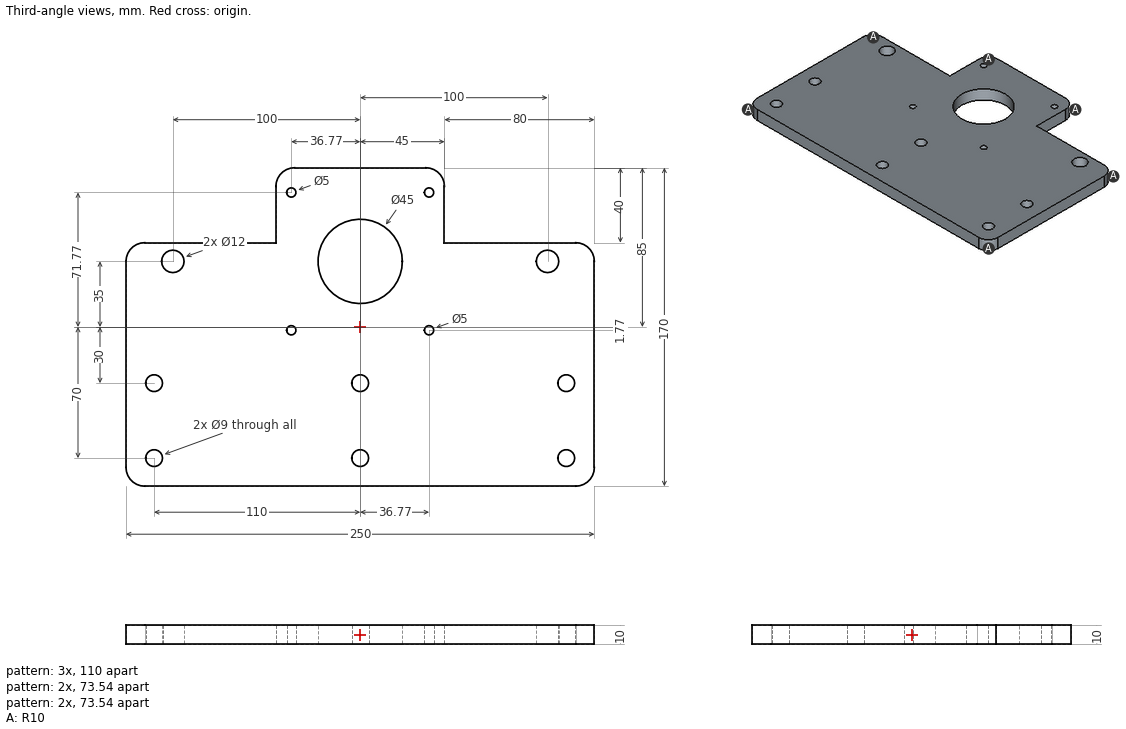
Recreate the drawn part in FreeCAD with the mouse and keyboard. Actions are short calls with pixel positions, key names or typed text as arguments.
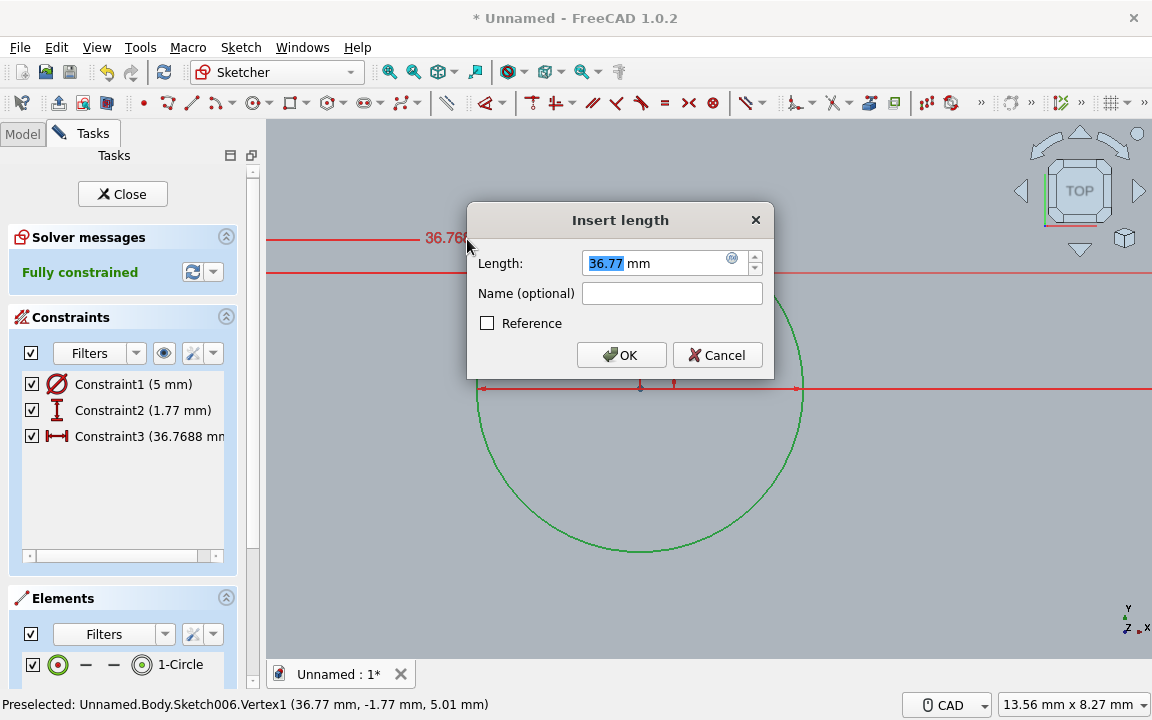
text(36.77)
key(Return)
key(Escape)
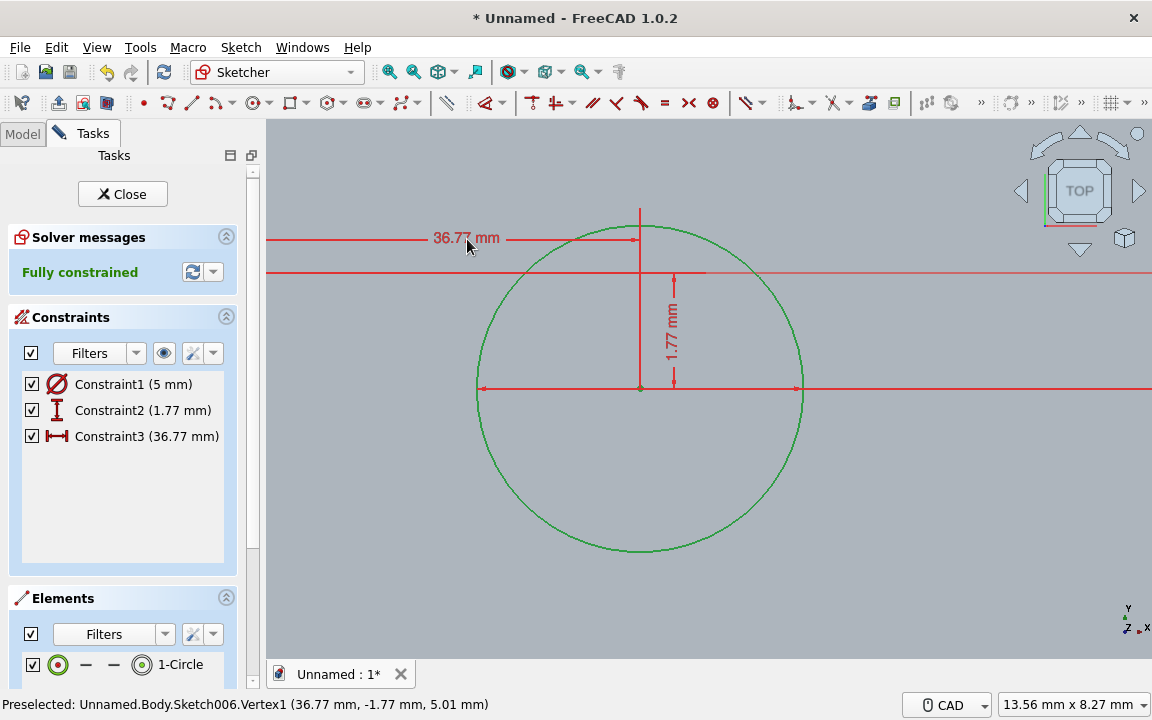
click(123, 194)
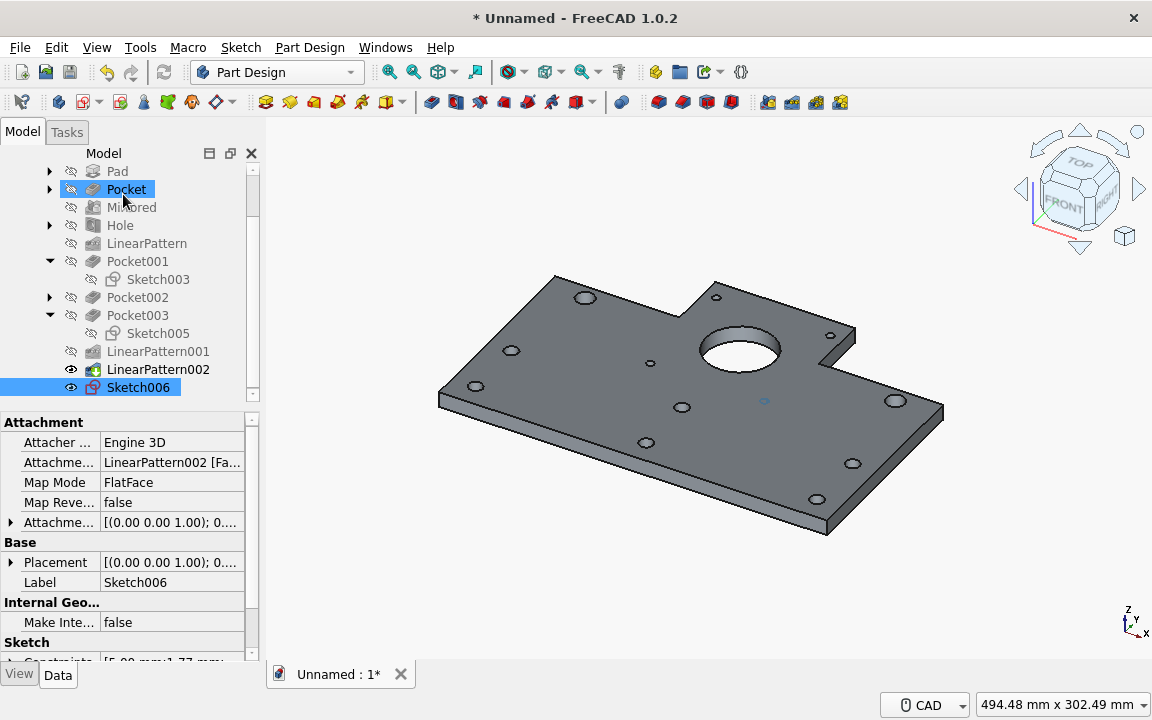
click(432, 102)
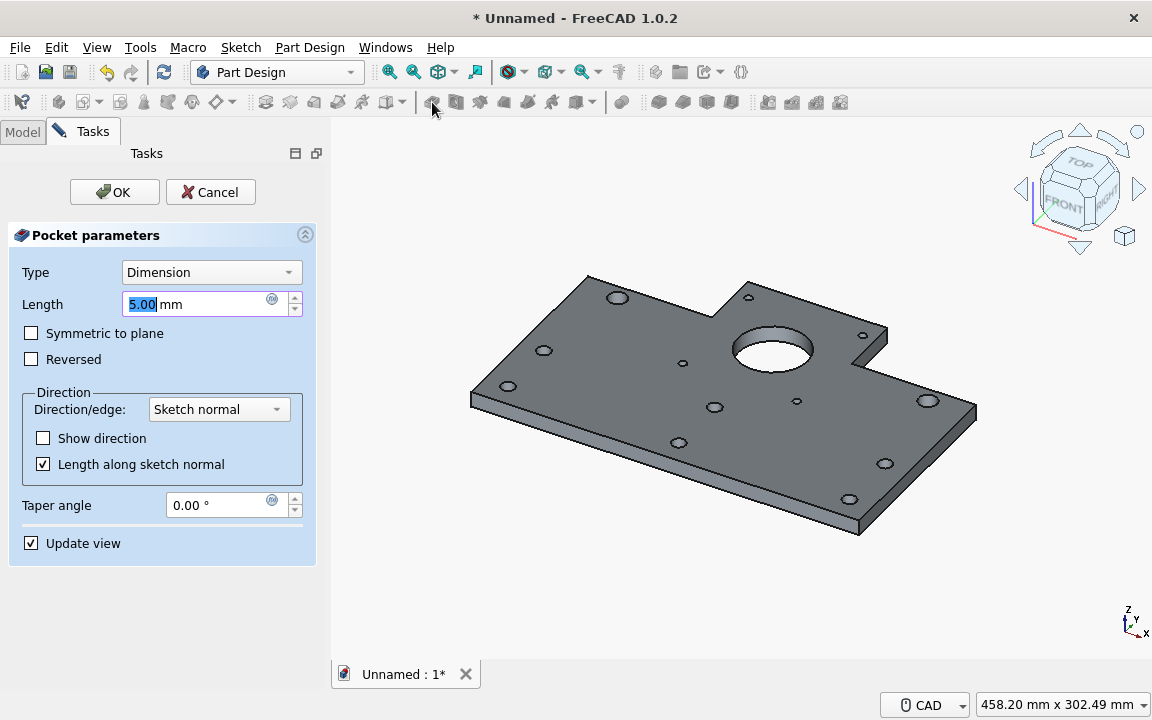
click(212, 272)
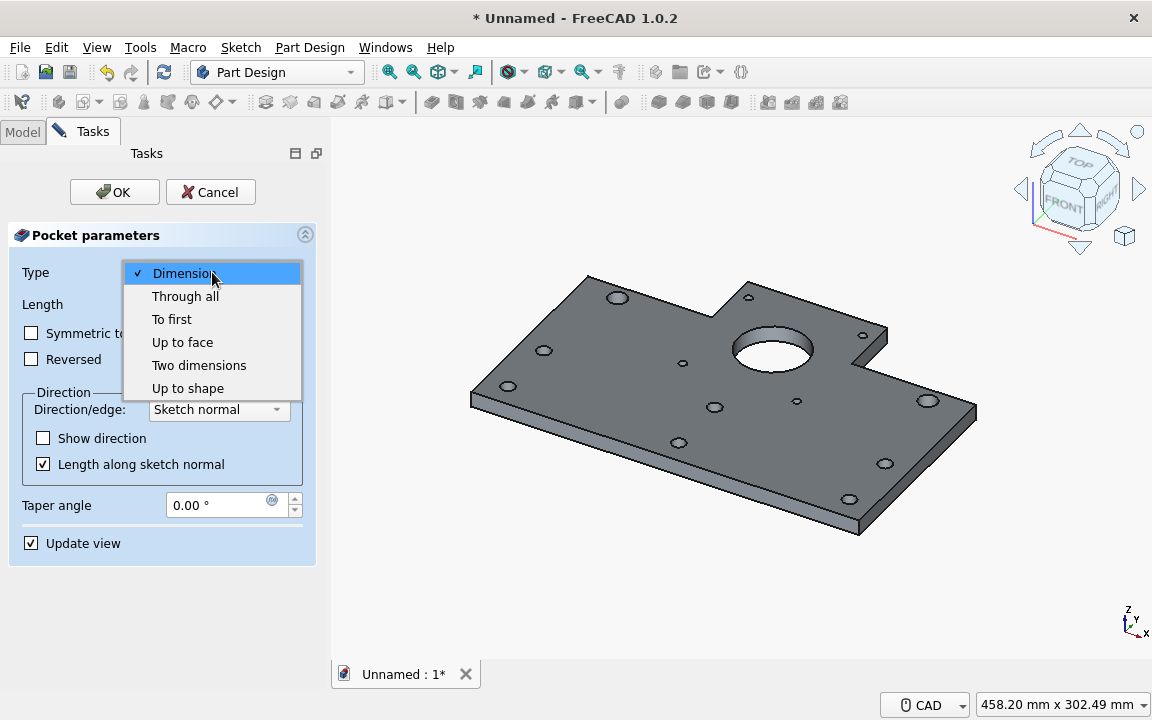
click(212, 296)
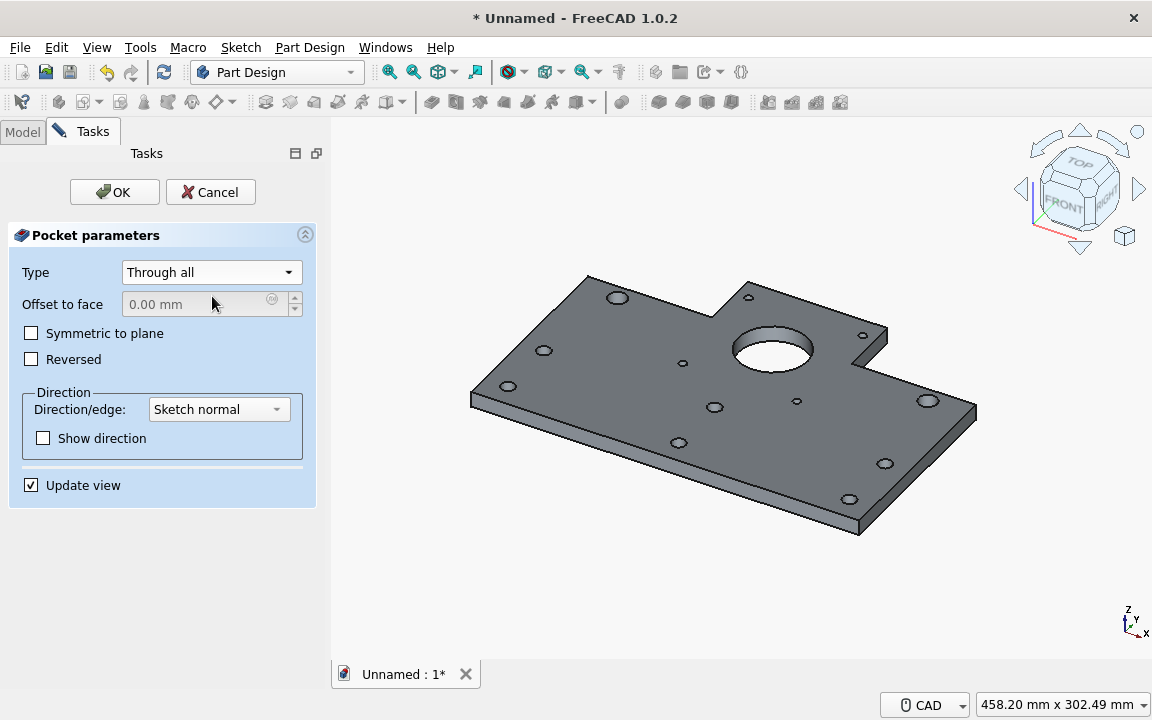
click(115, 192)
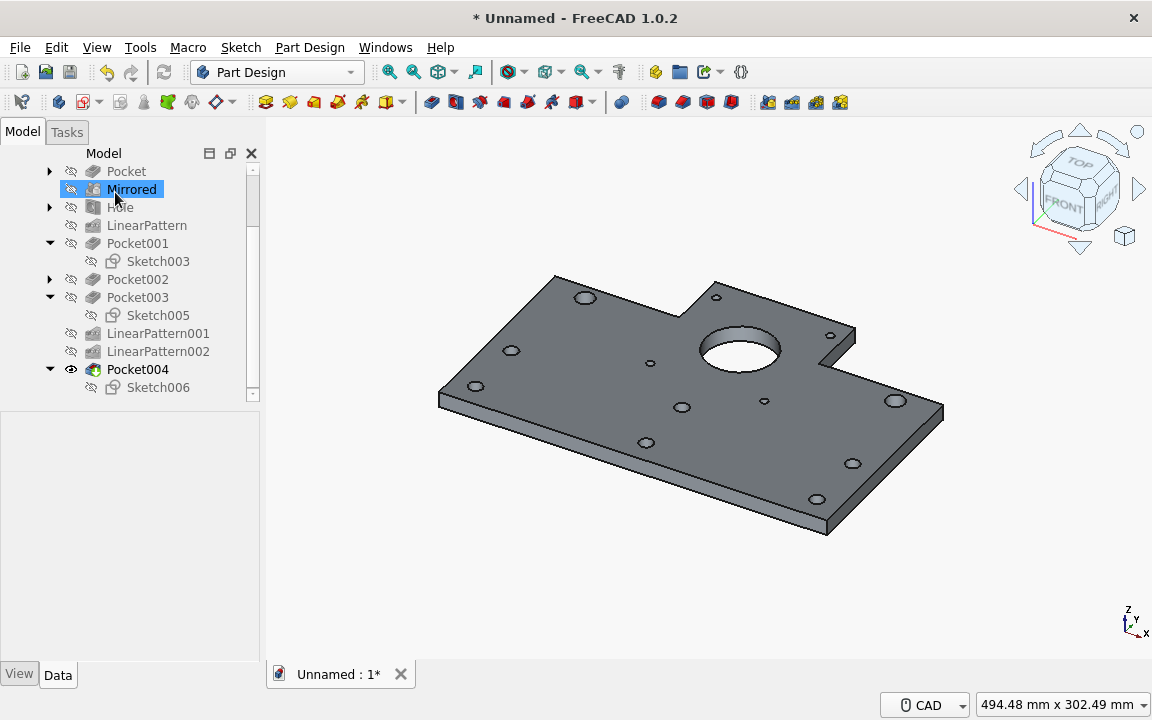
click(827, 527)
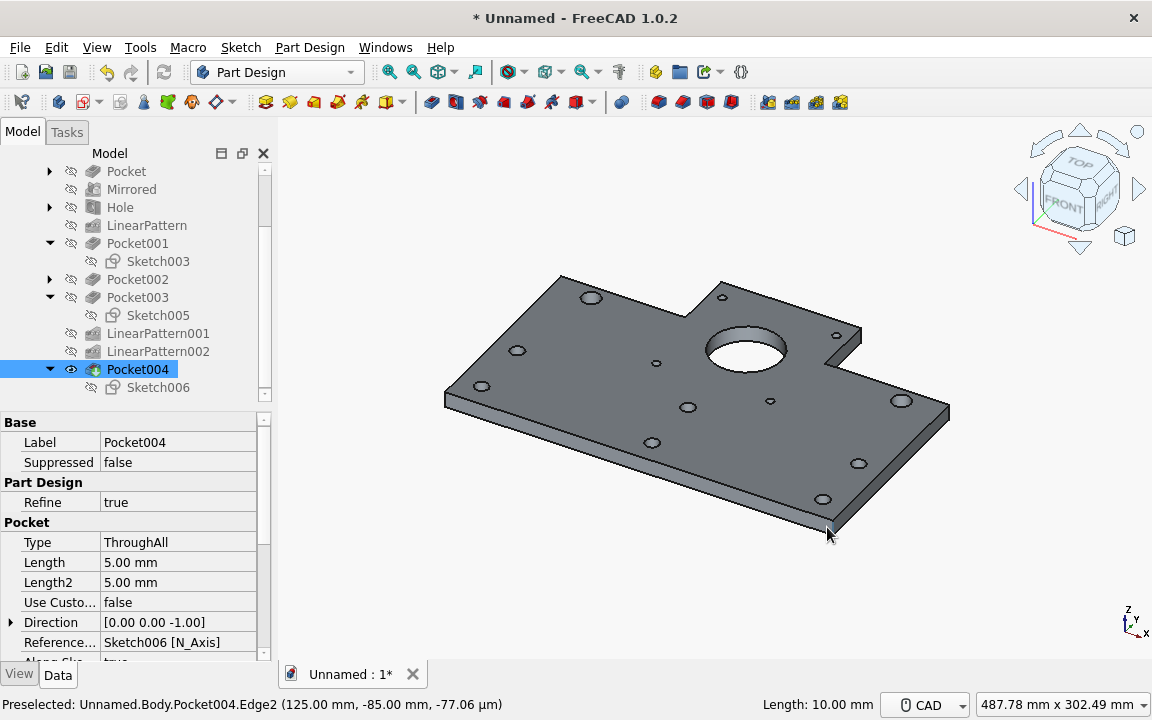
scroll(949, 411, up, 5)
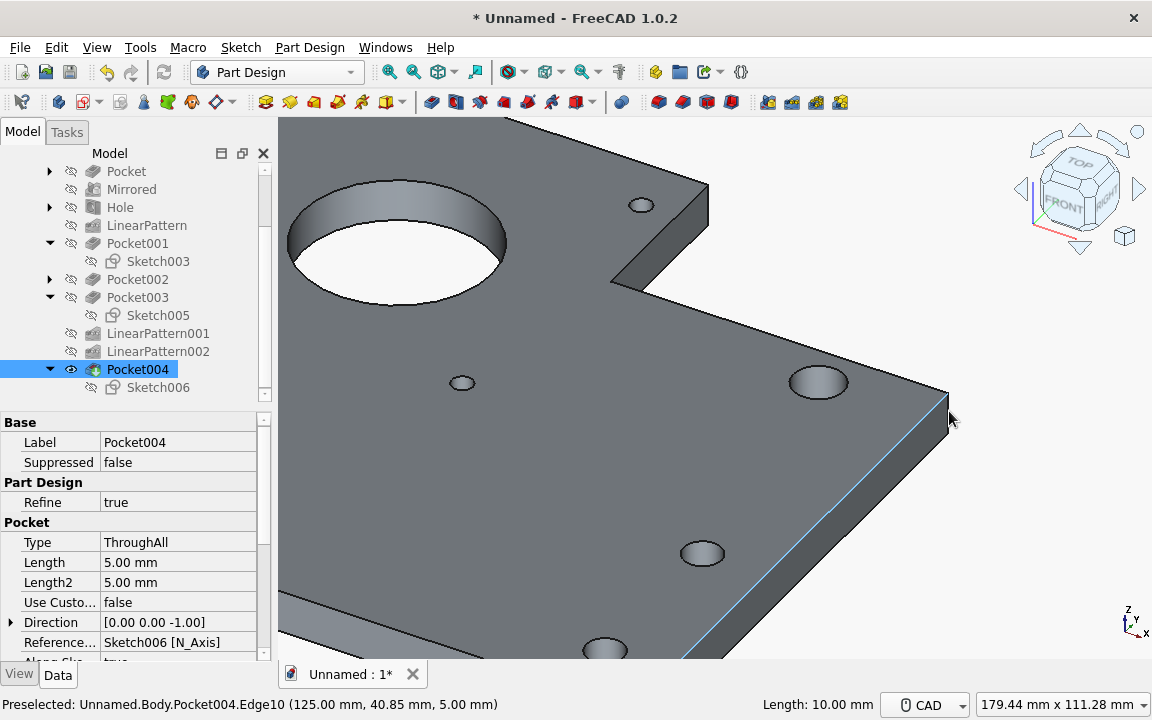
click(390, 72)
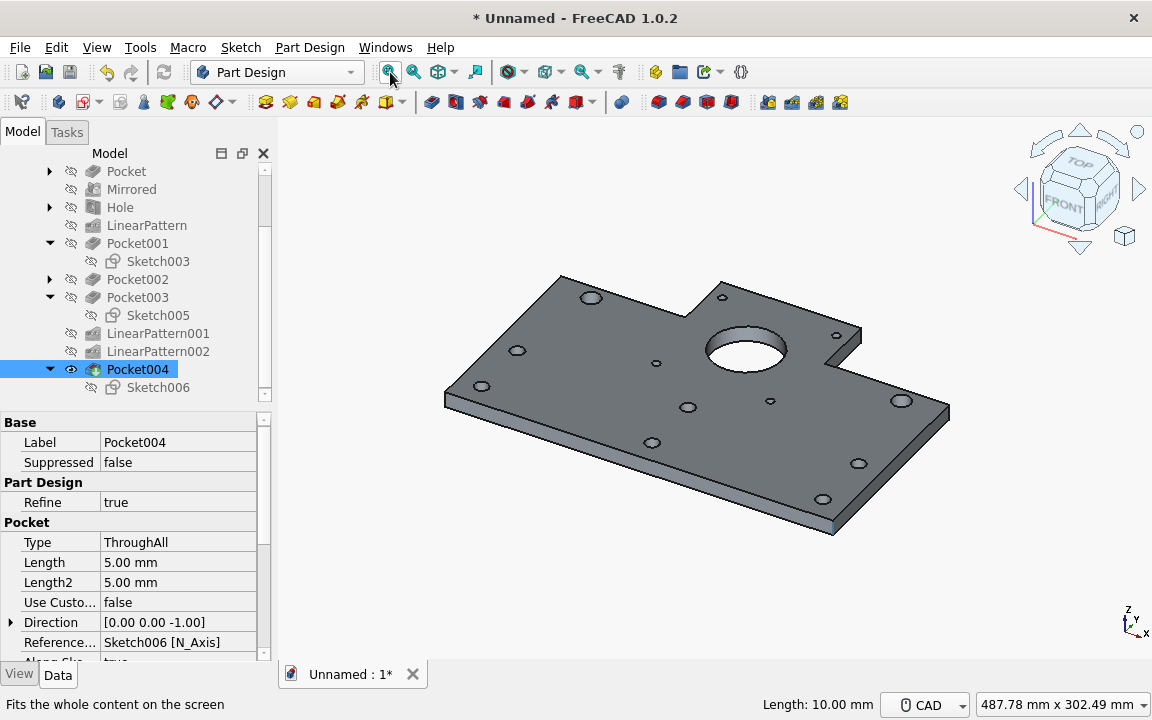
key(0)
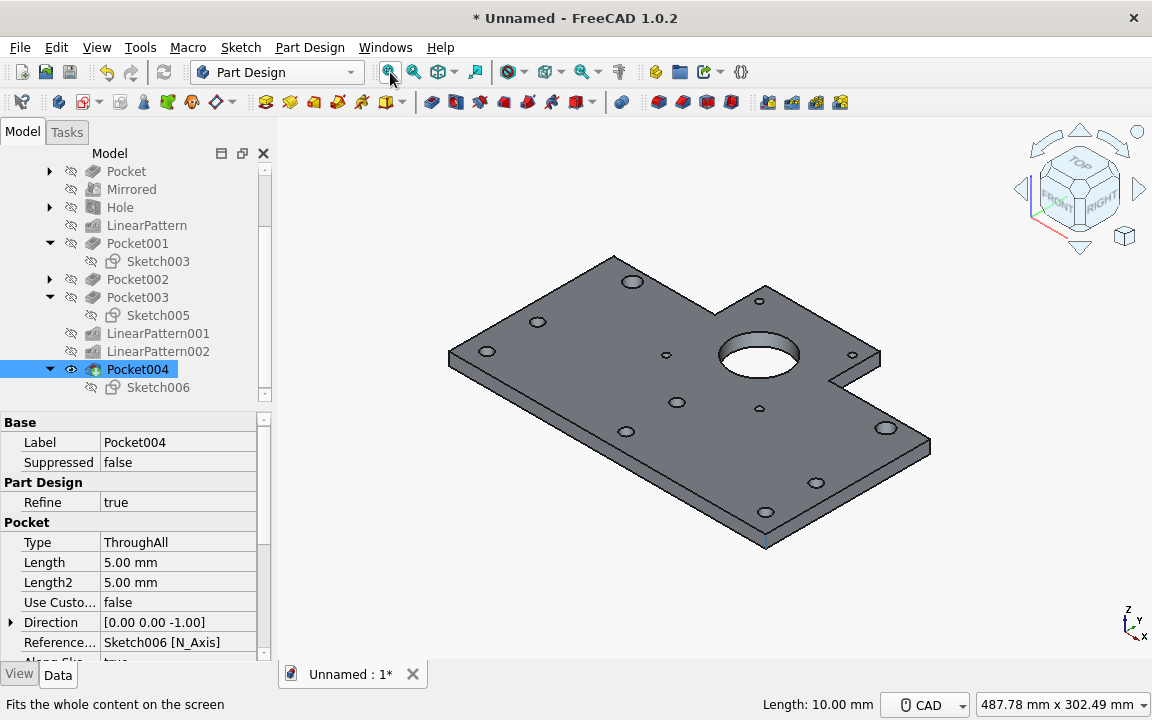
scroll(930, 446, up, 5)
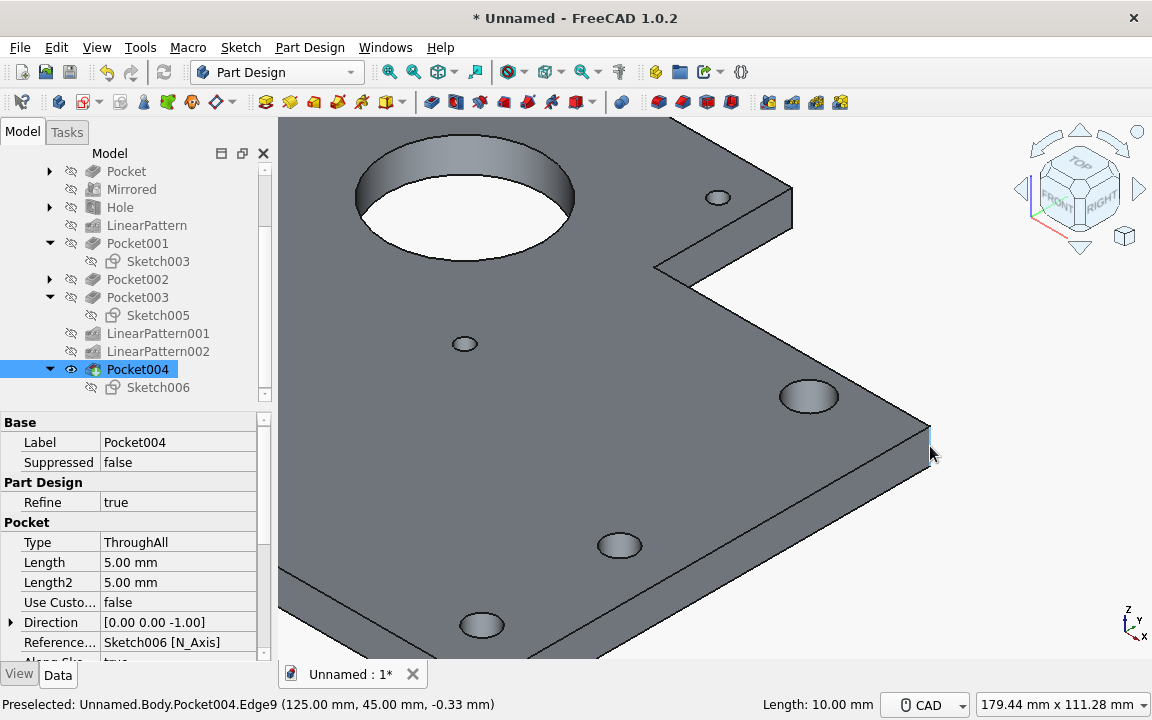
key(v)
key(f)